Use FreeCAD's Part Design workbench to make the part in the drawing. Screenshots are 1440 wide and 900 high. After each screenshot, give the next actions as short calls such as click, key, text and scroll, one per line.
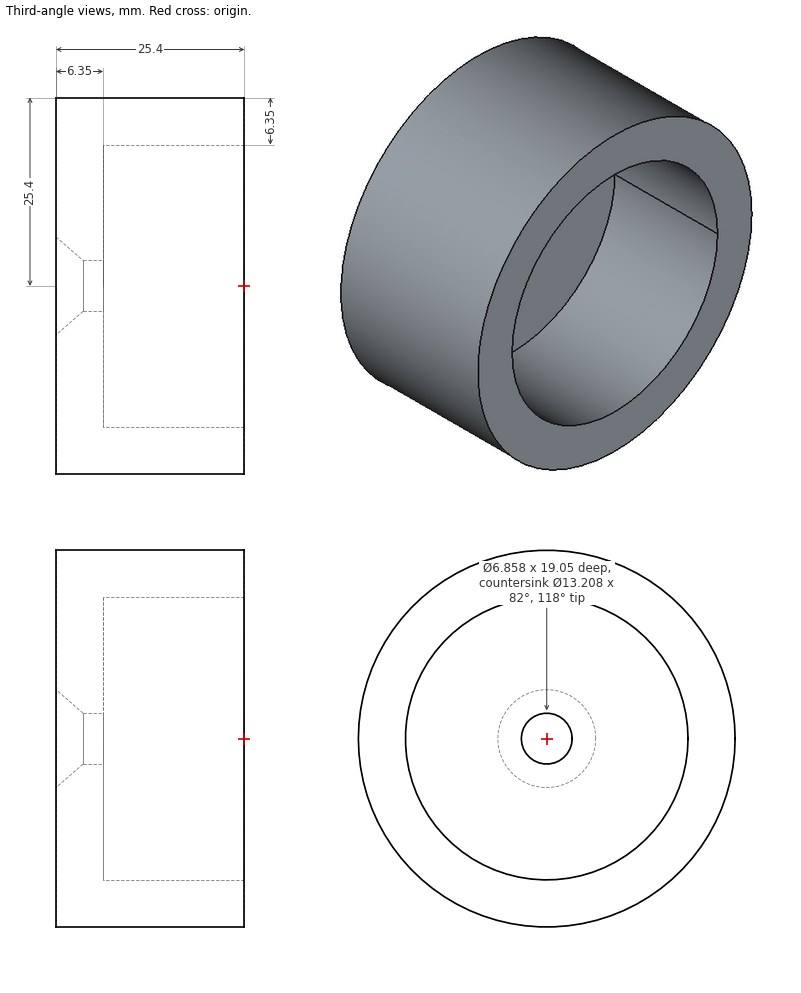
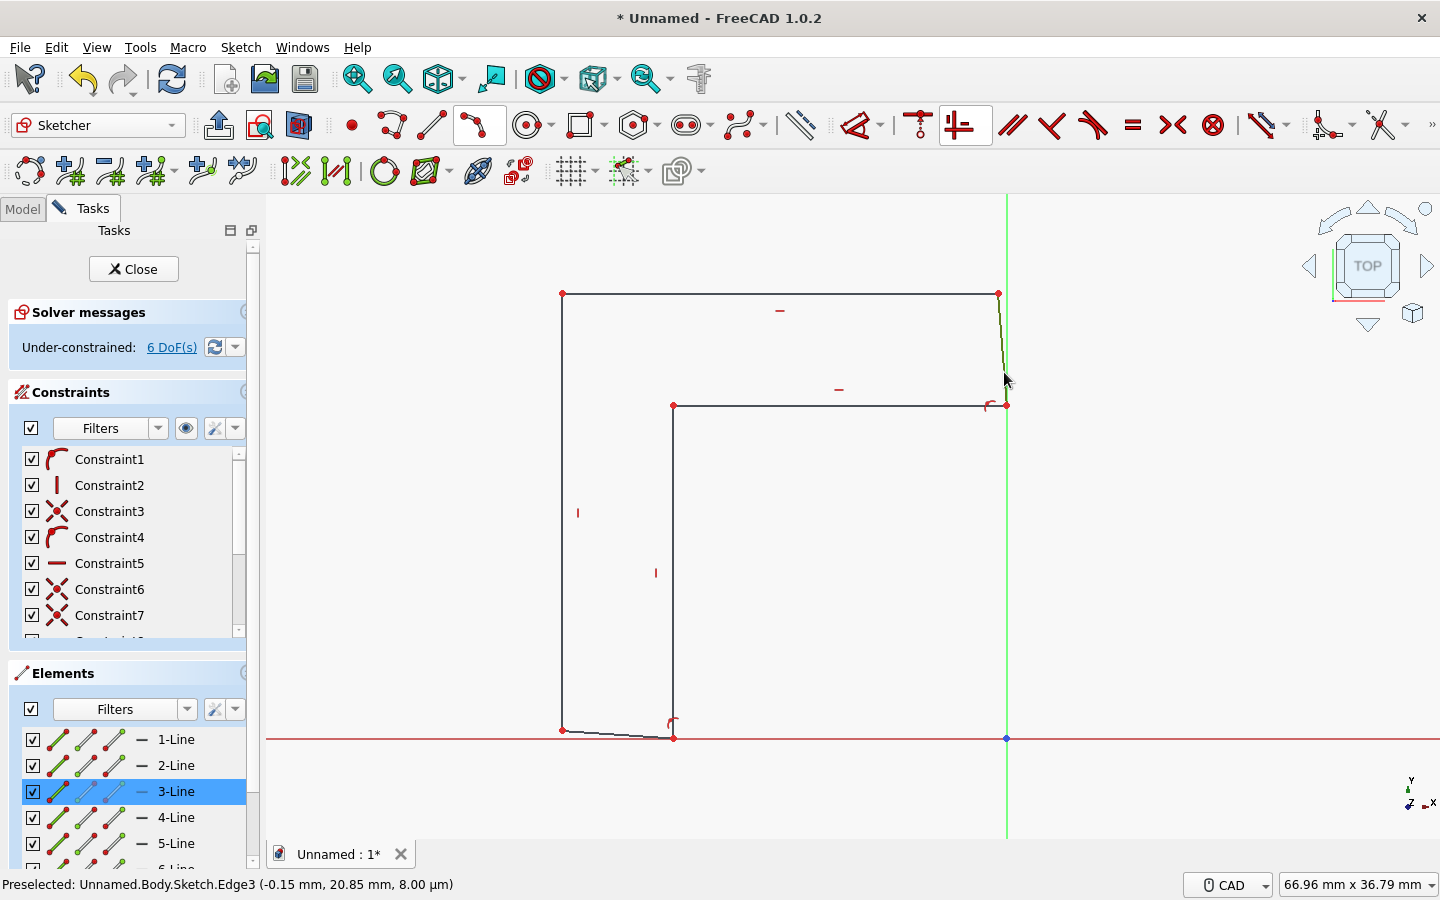
click(986, 126)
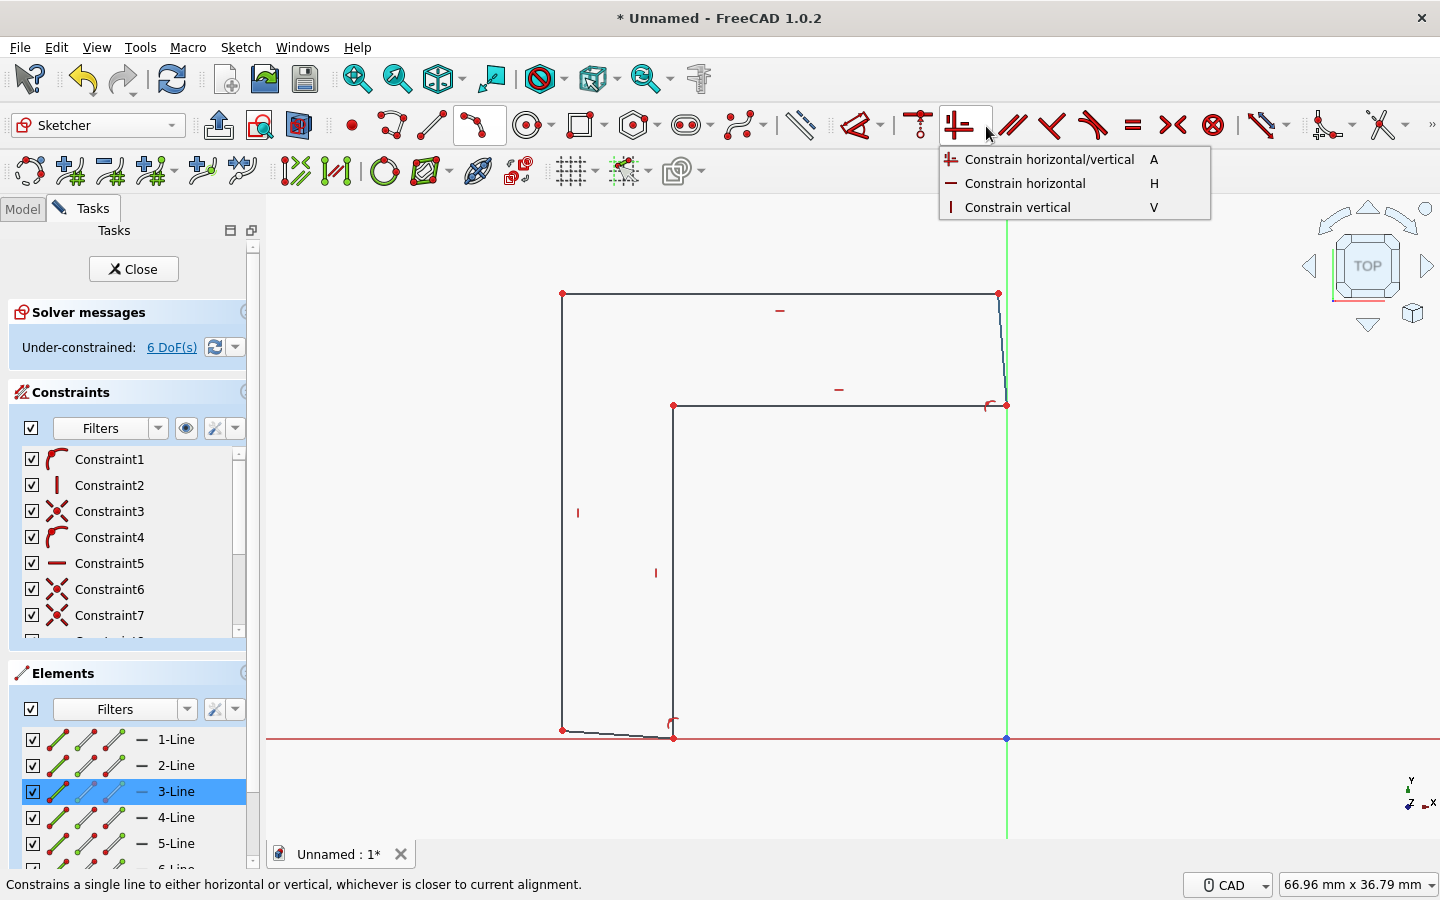
click(1075, 207)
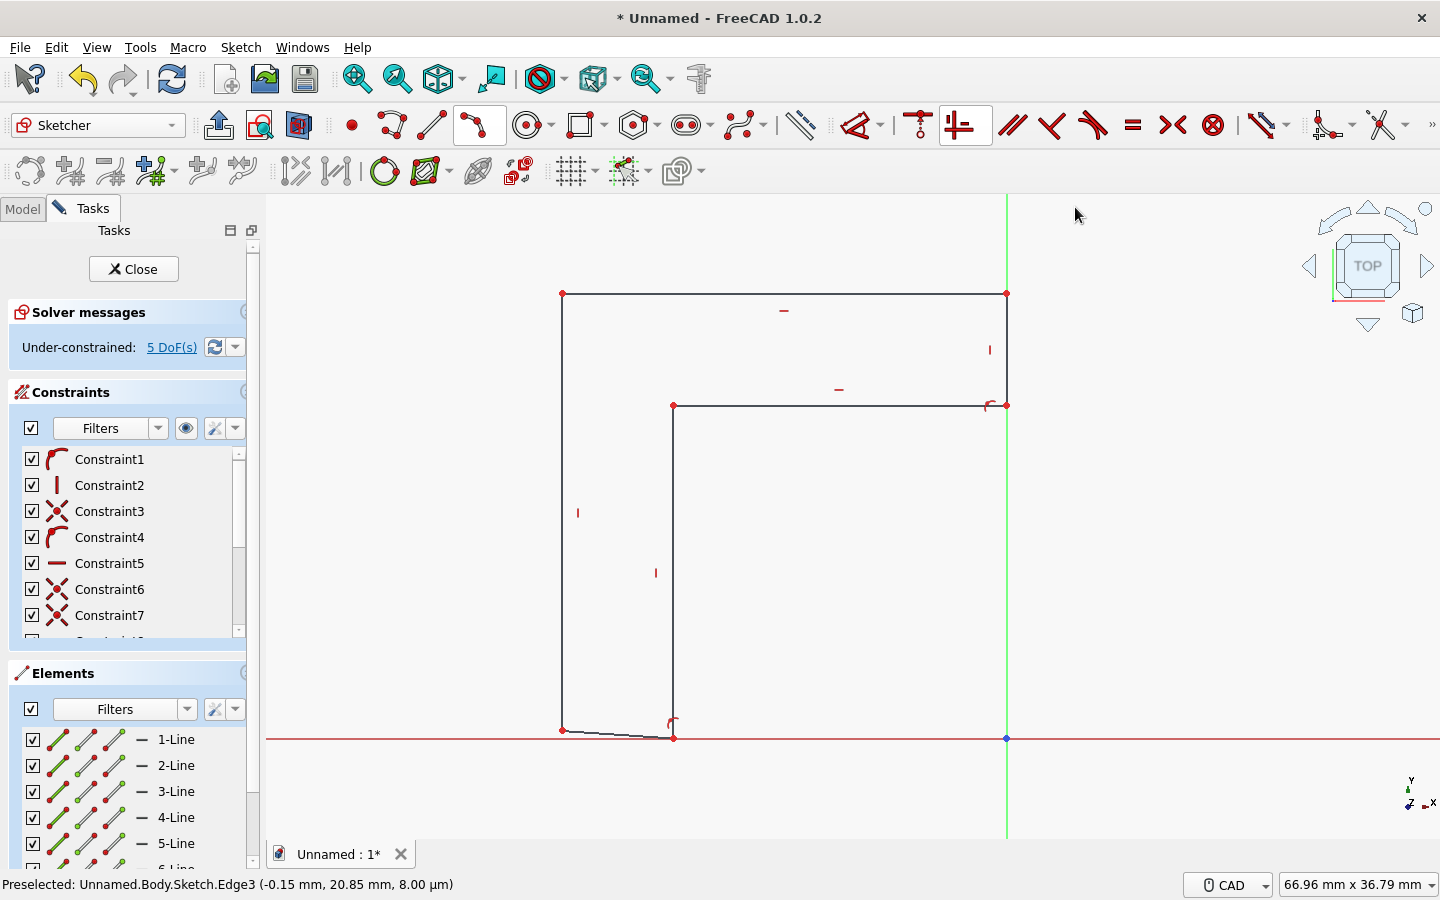
click(640, 736)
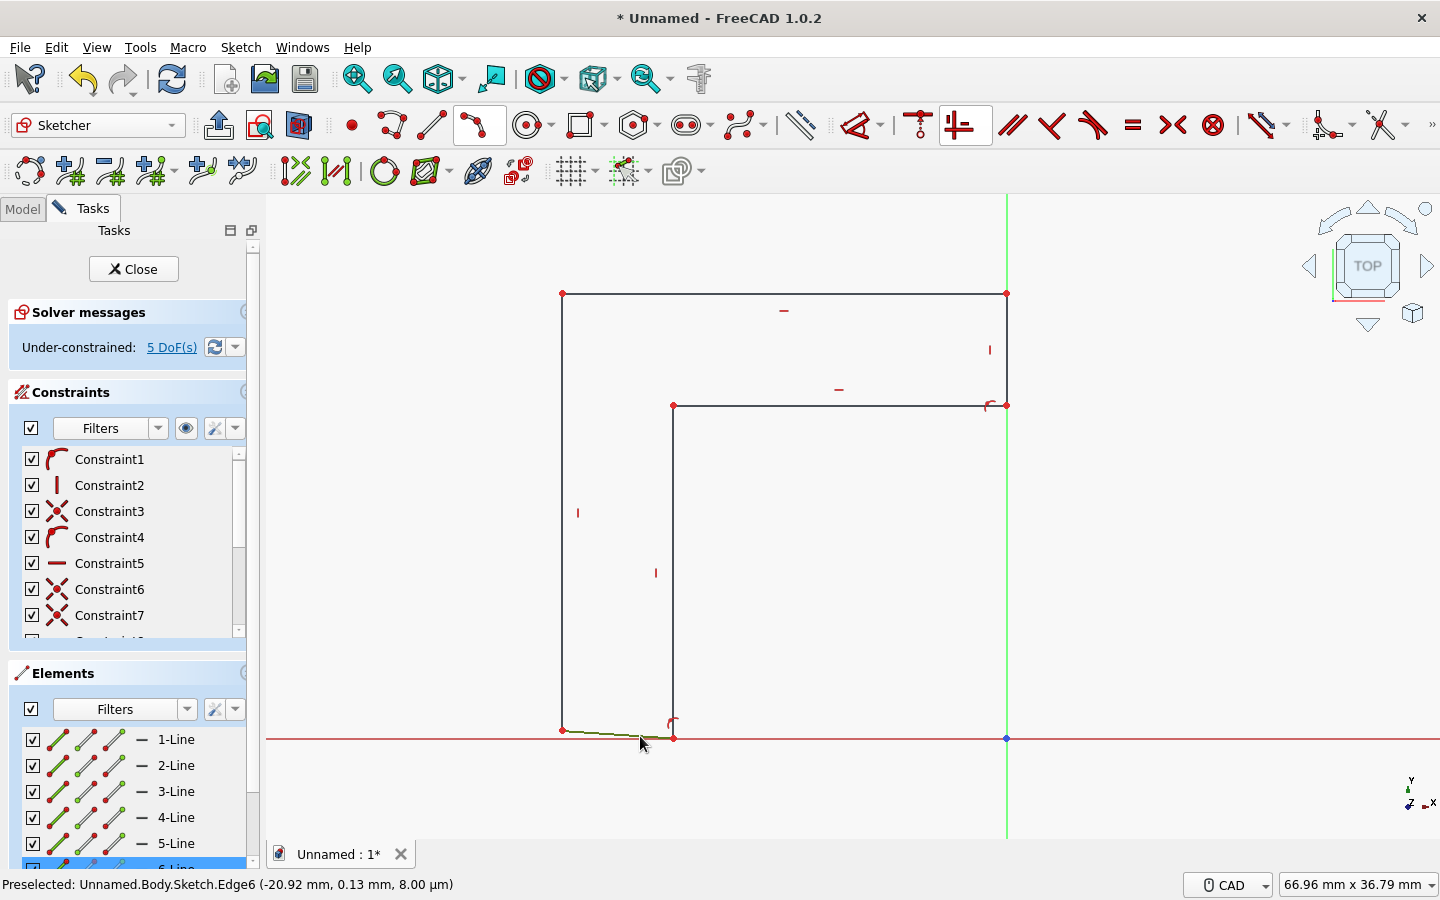
key(h)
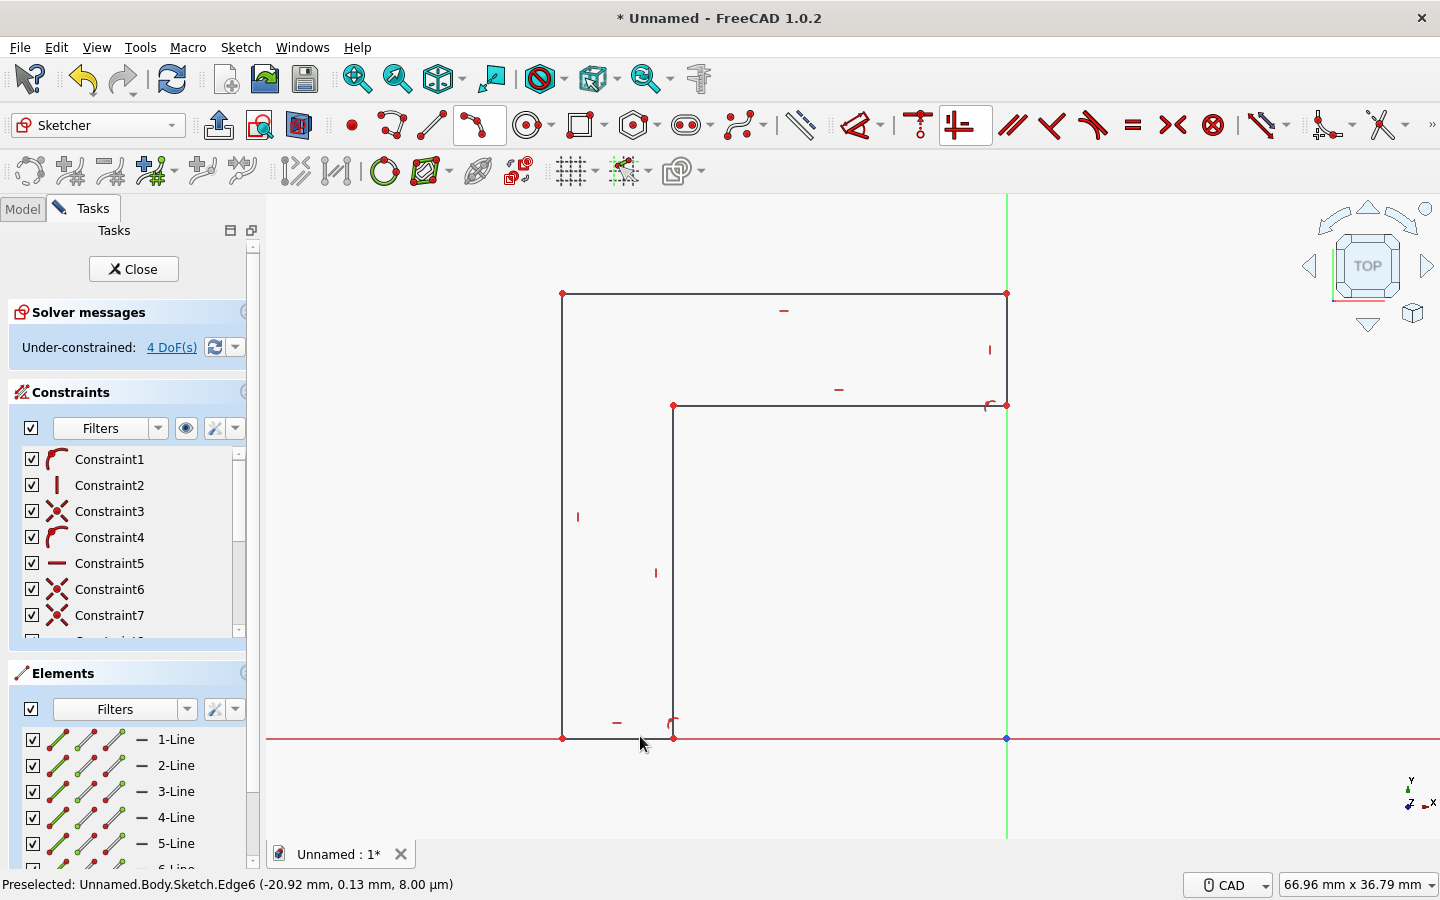
click(856, 126)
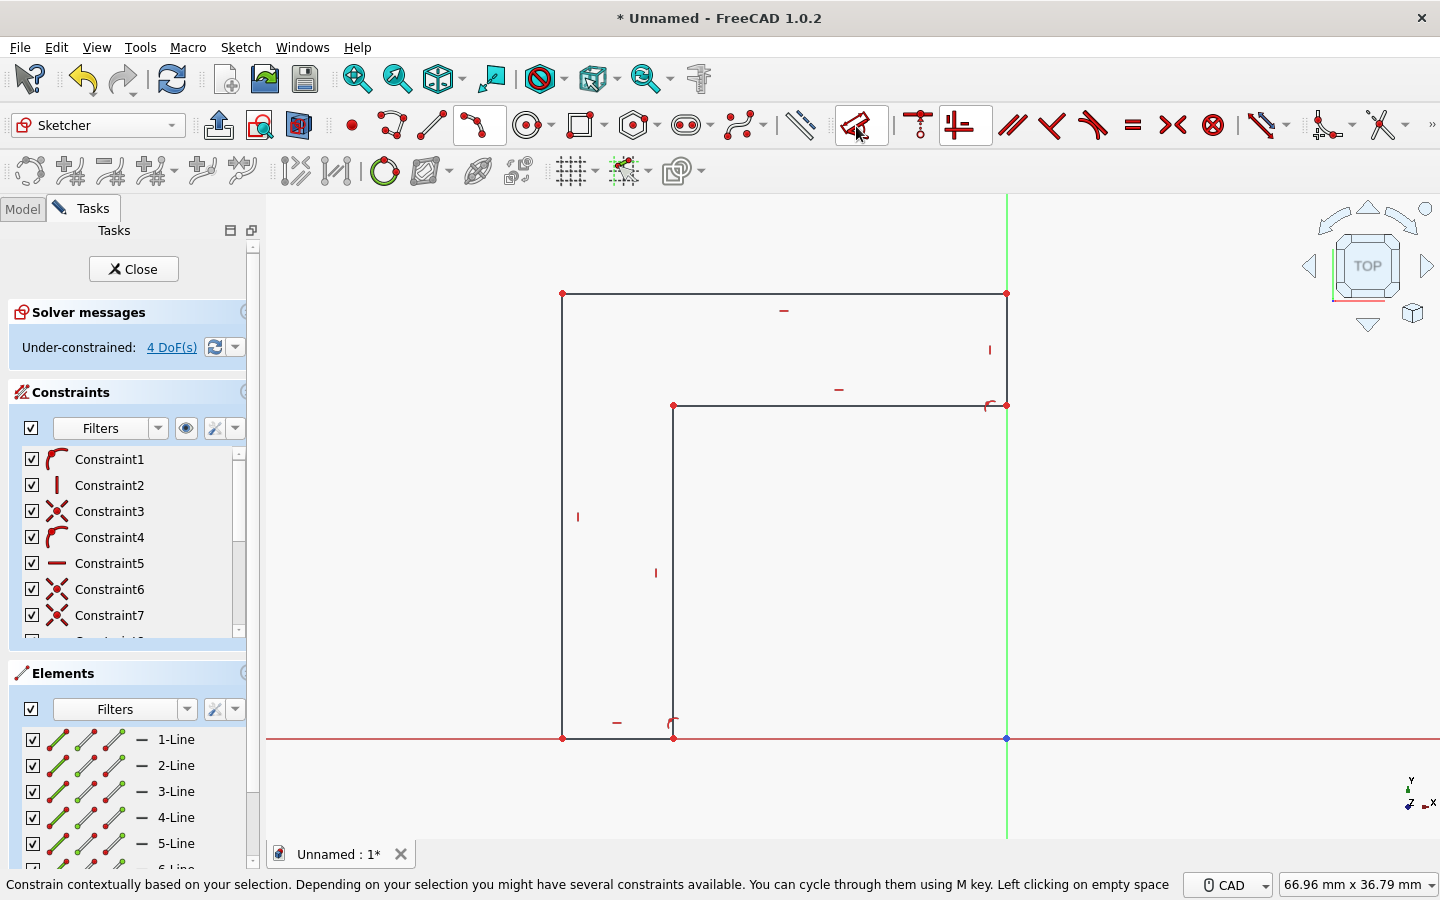
click(1007, 372)
click(1041, 350)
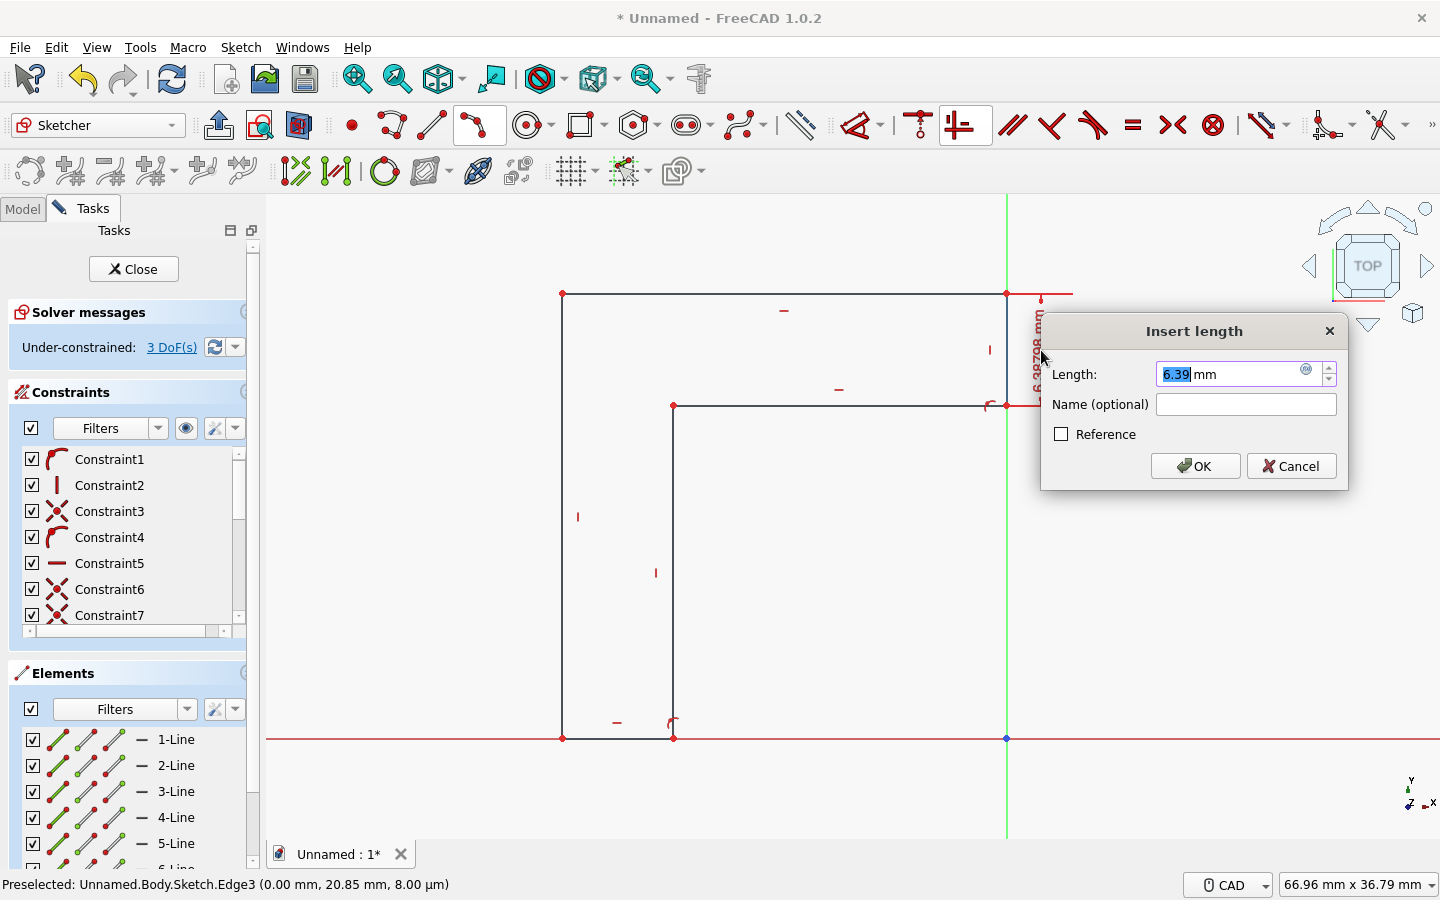
text(6.35)
key(Return)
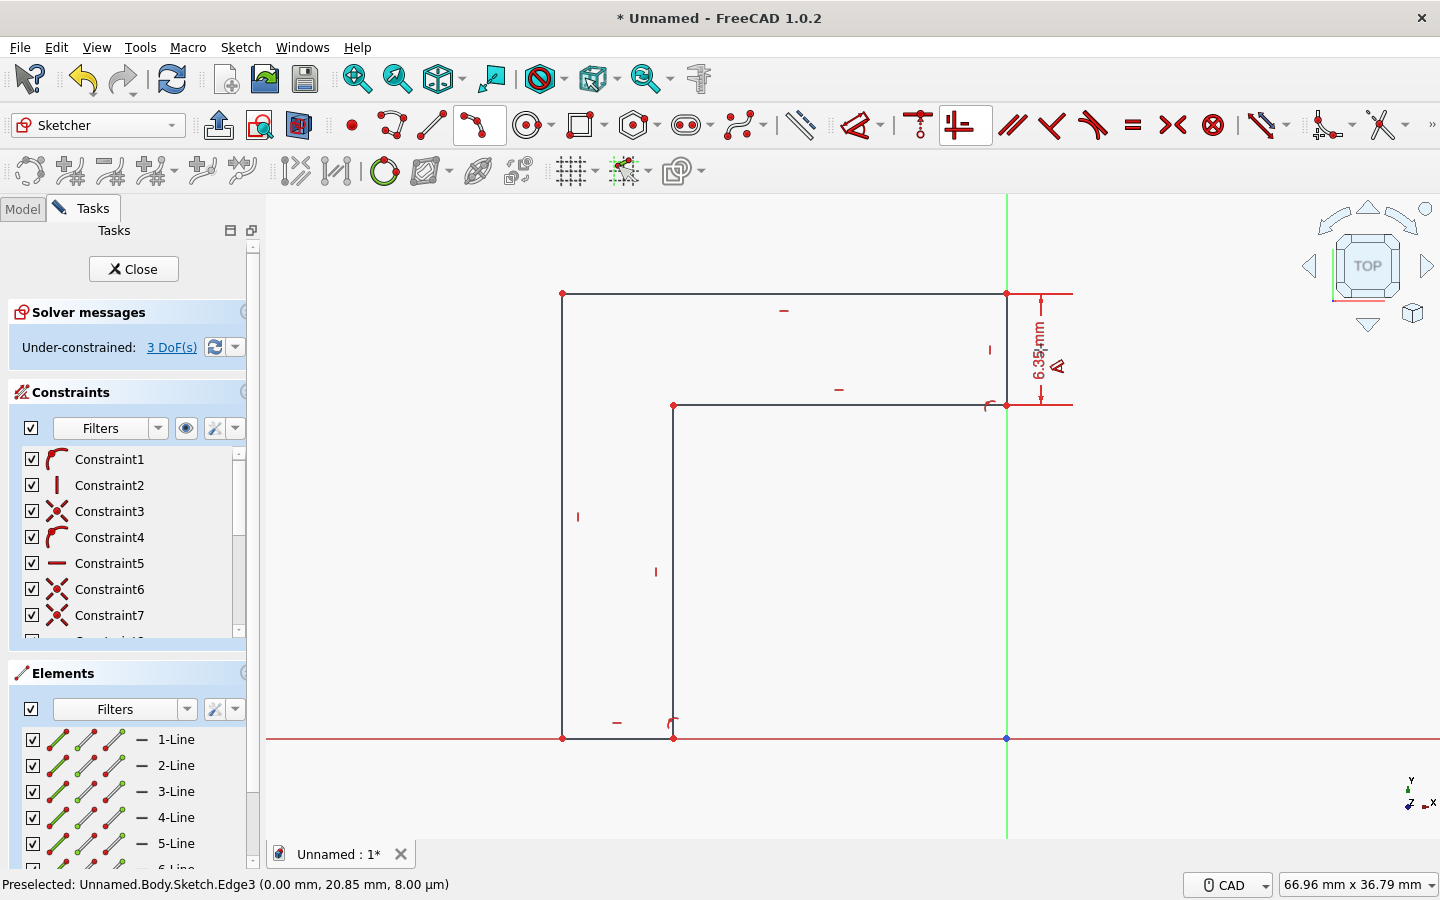
click(873, 294)
click(784, 260)